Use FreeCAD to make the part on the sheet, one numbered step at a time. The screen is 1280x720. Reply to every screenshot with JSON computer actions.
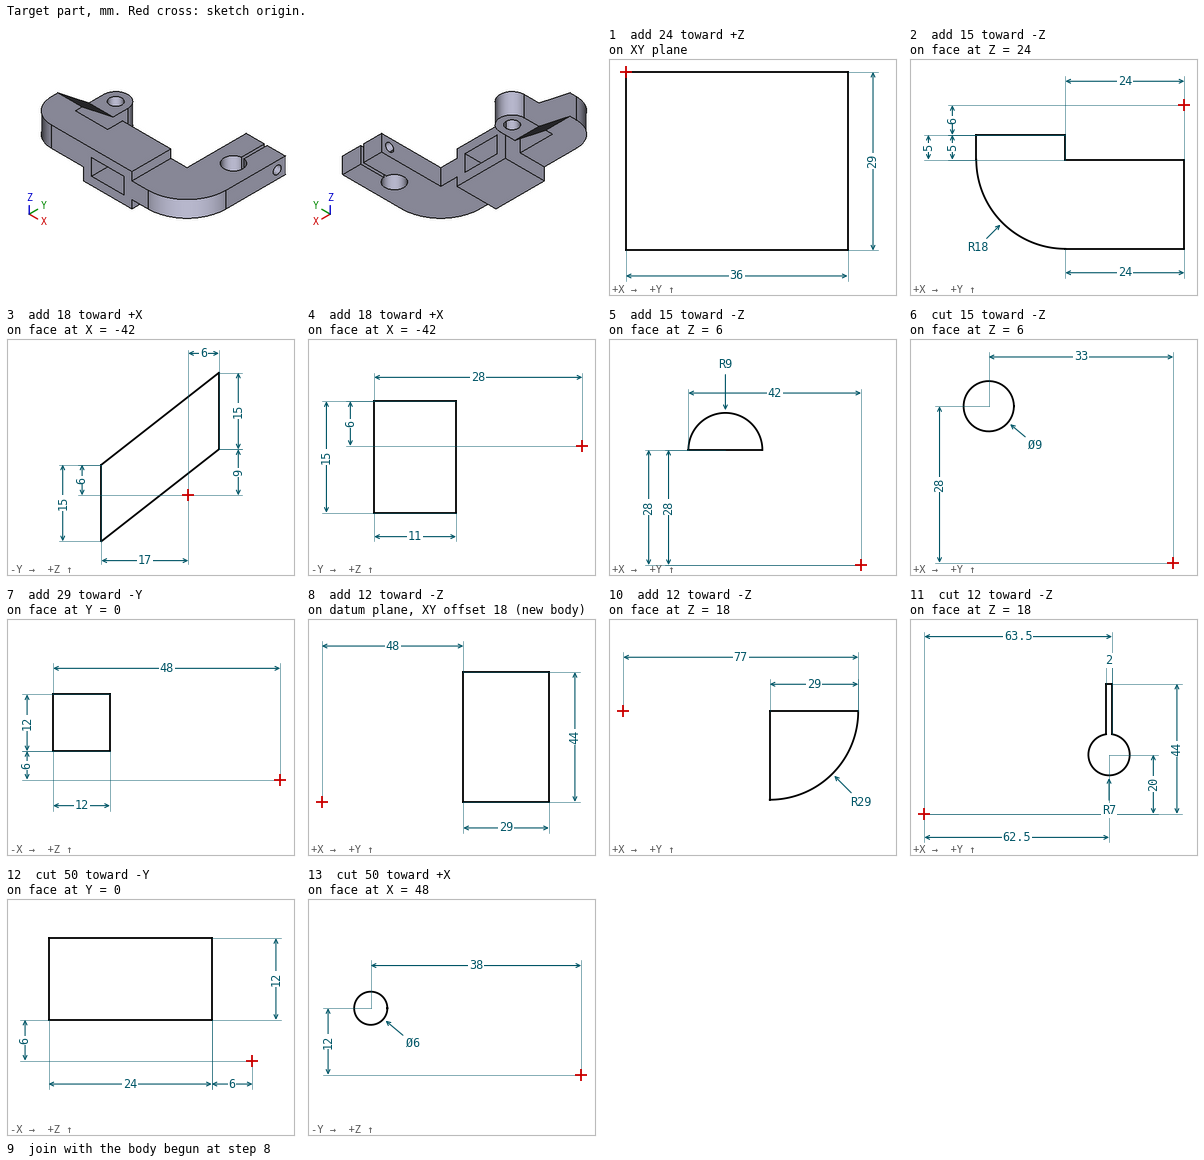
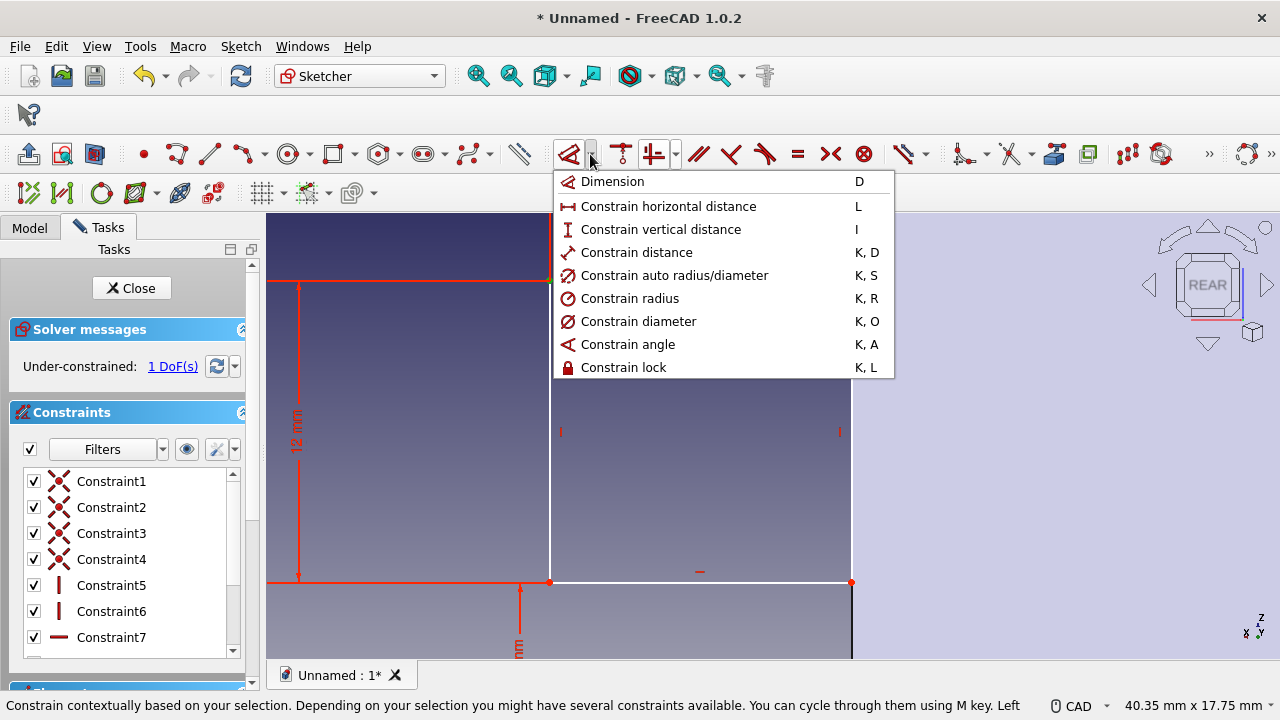
{"action": "left_click", "coordinate": [724, 206]}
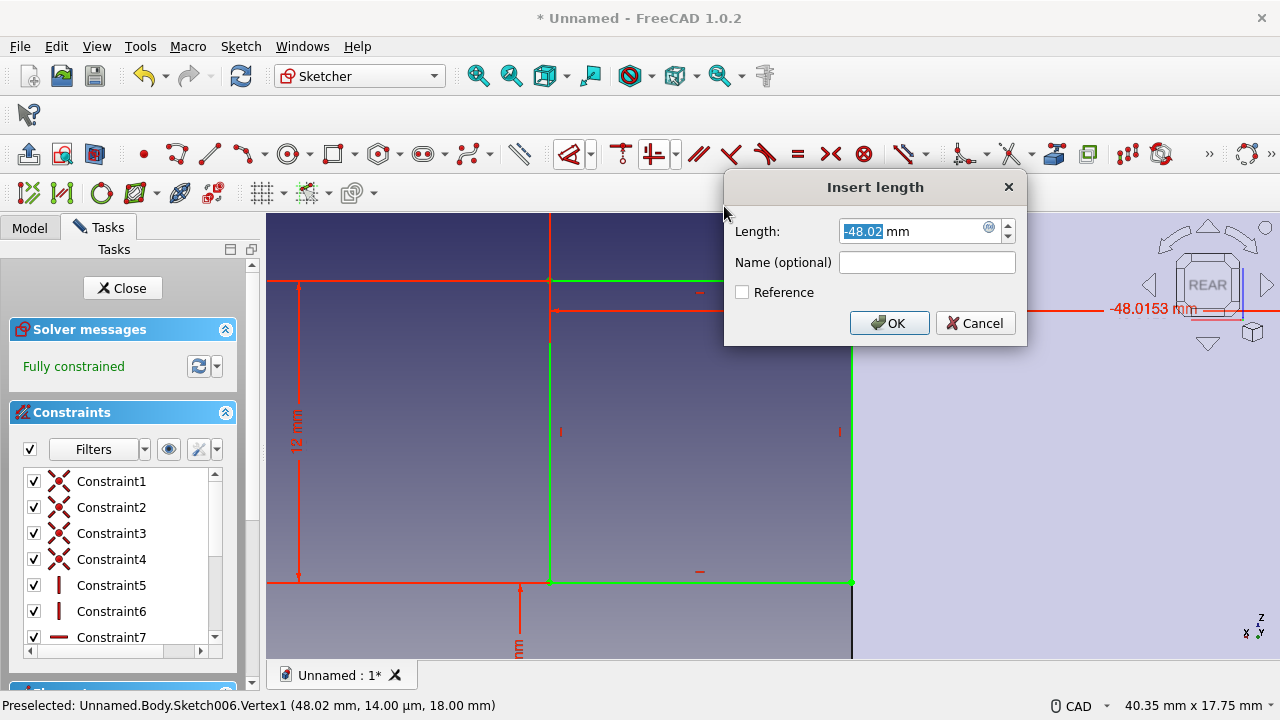
{"action": "type", "text": "-48"}
{"action": "key", "text": "Return"}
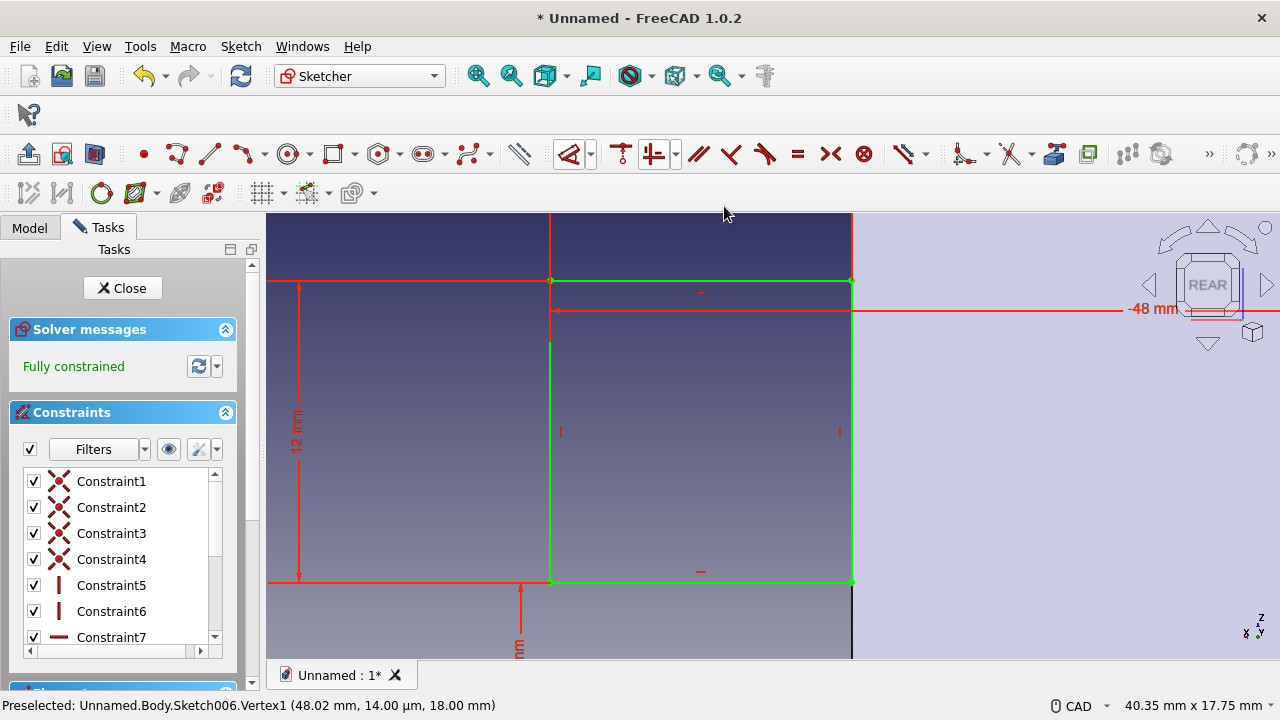
{"action": "left_click", "coordinate": [123, 288]}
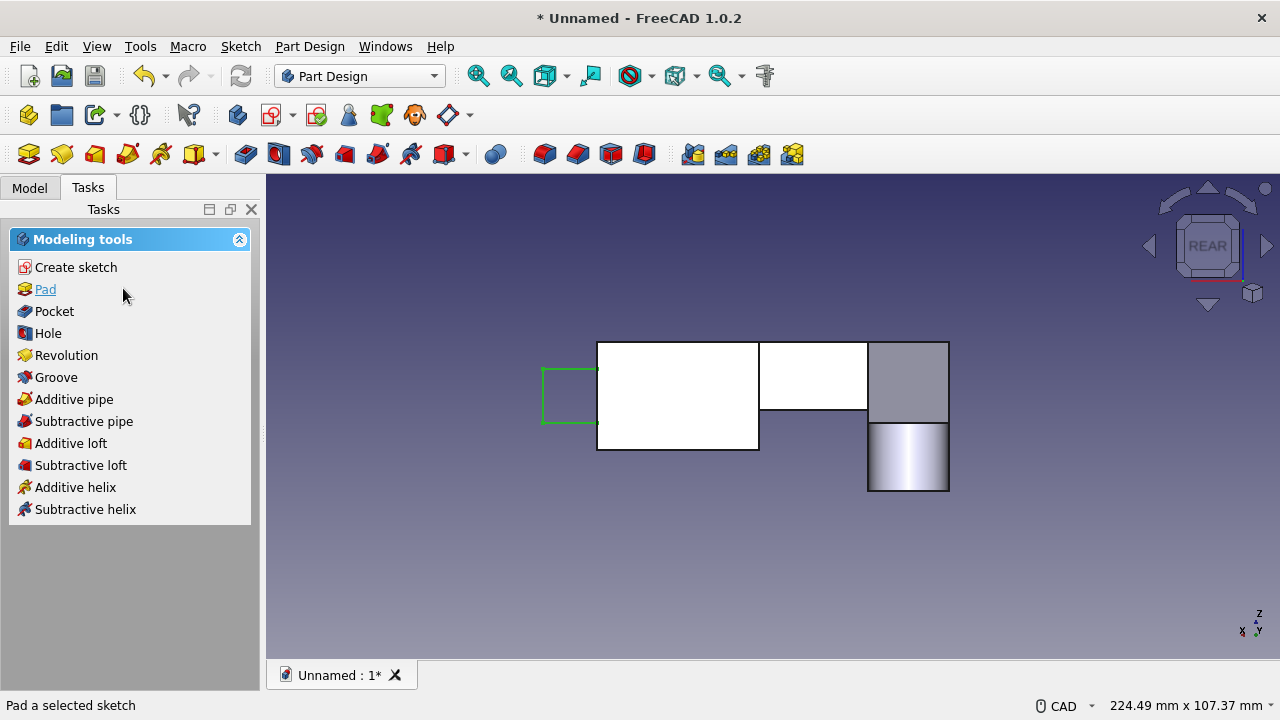
{"action": "left_click", "coordinate": [29, 154]}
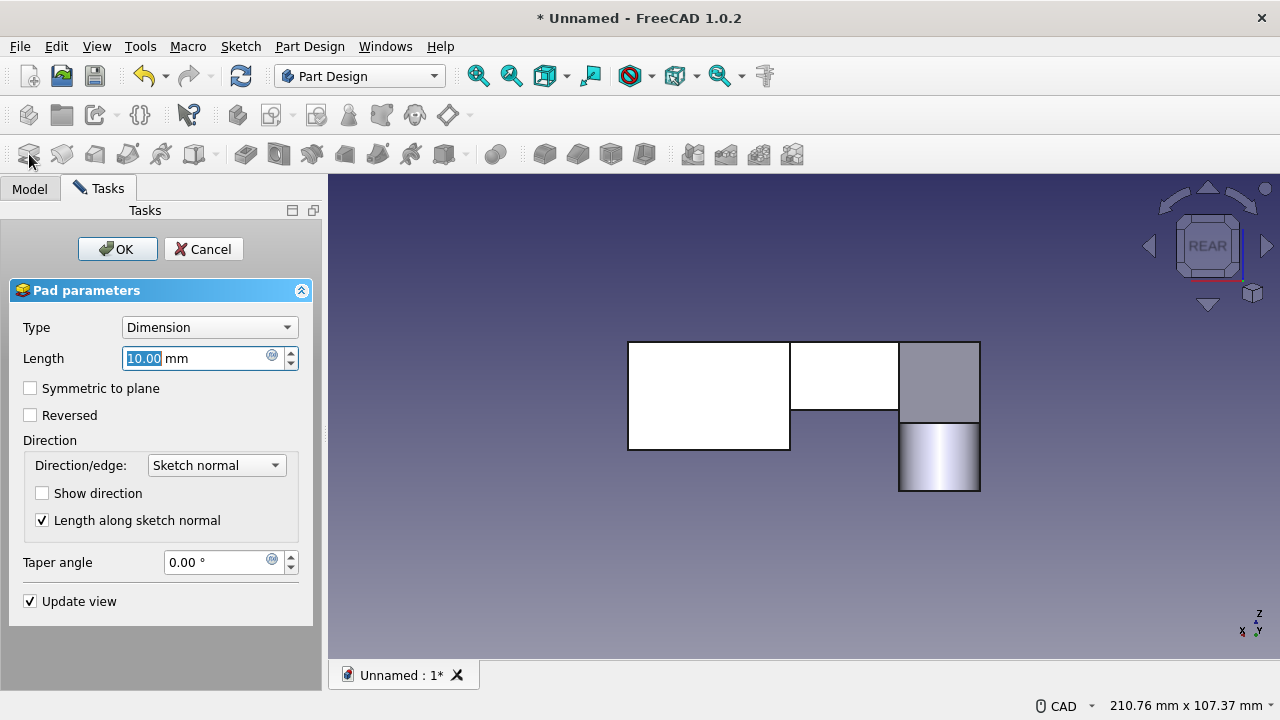
{"action": "type", "text": "29"}
{"action": "key", "text": "Tab"}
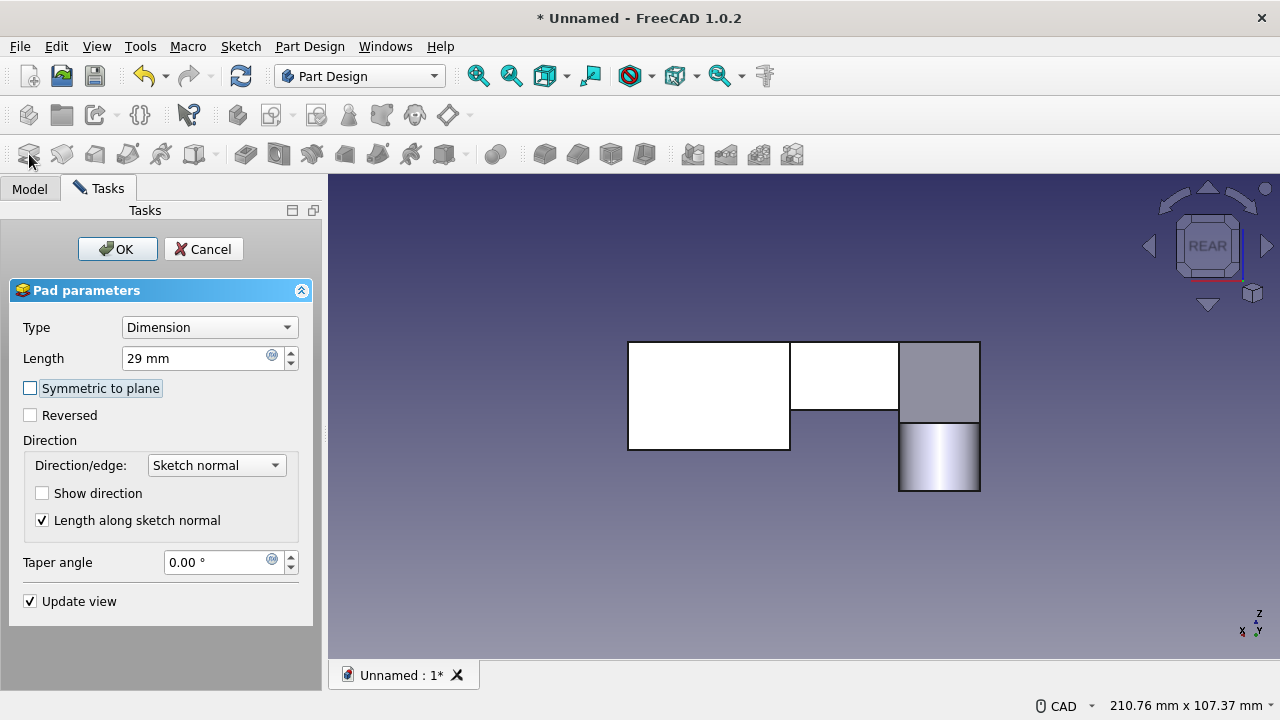
{"action": "left_click", "coordinate": [31, 415]}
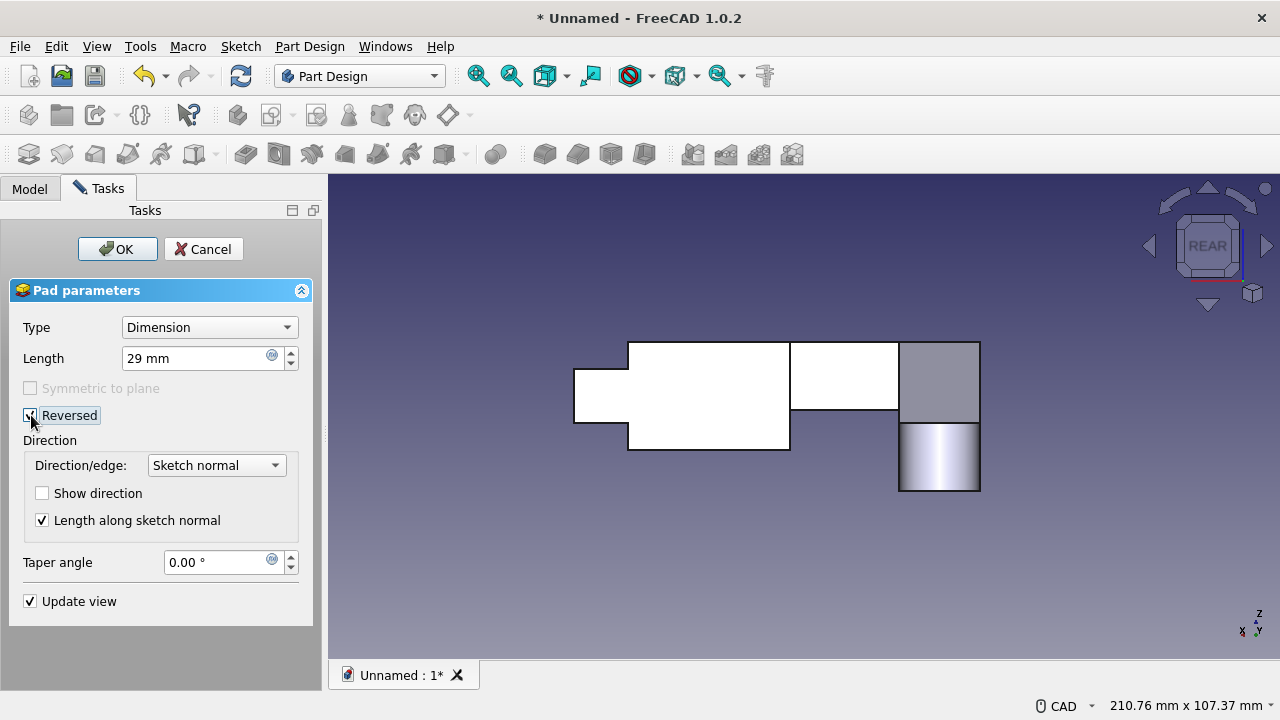
{"action": "left_click", "coordinate": [118, 249]}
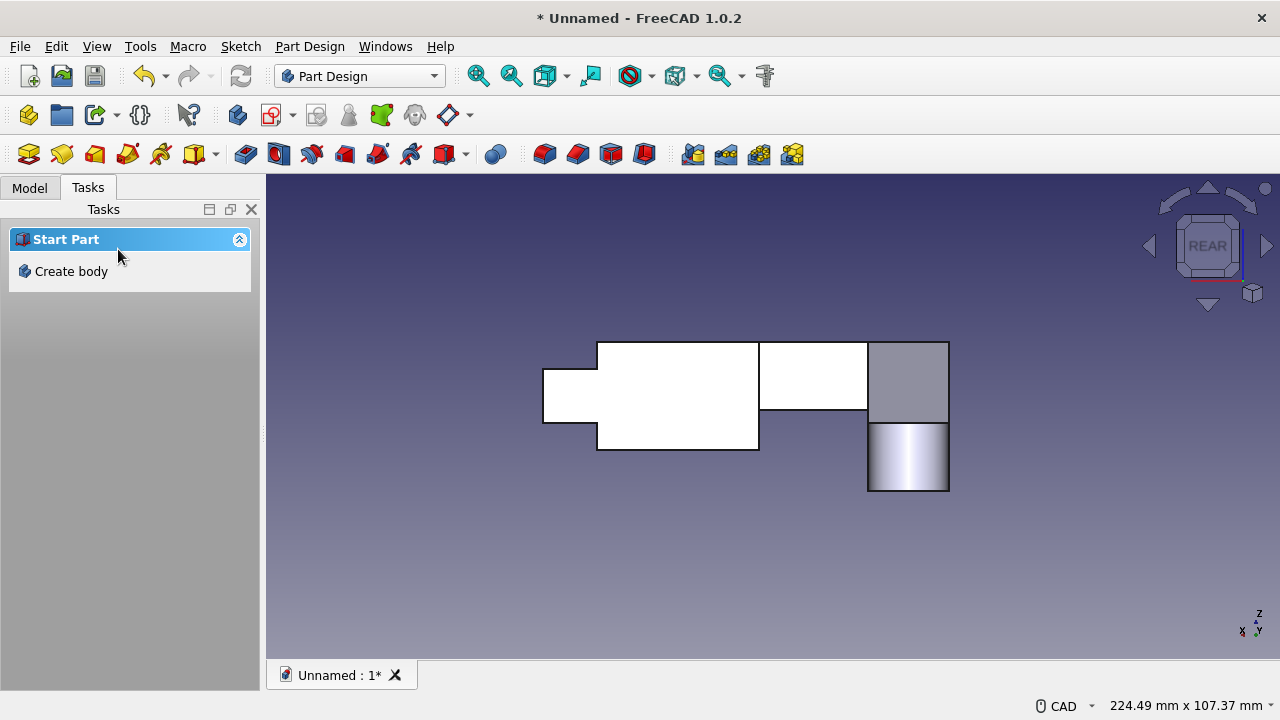
{"action": "key", "text": "v f"}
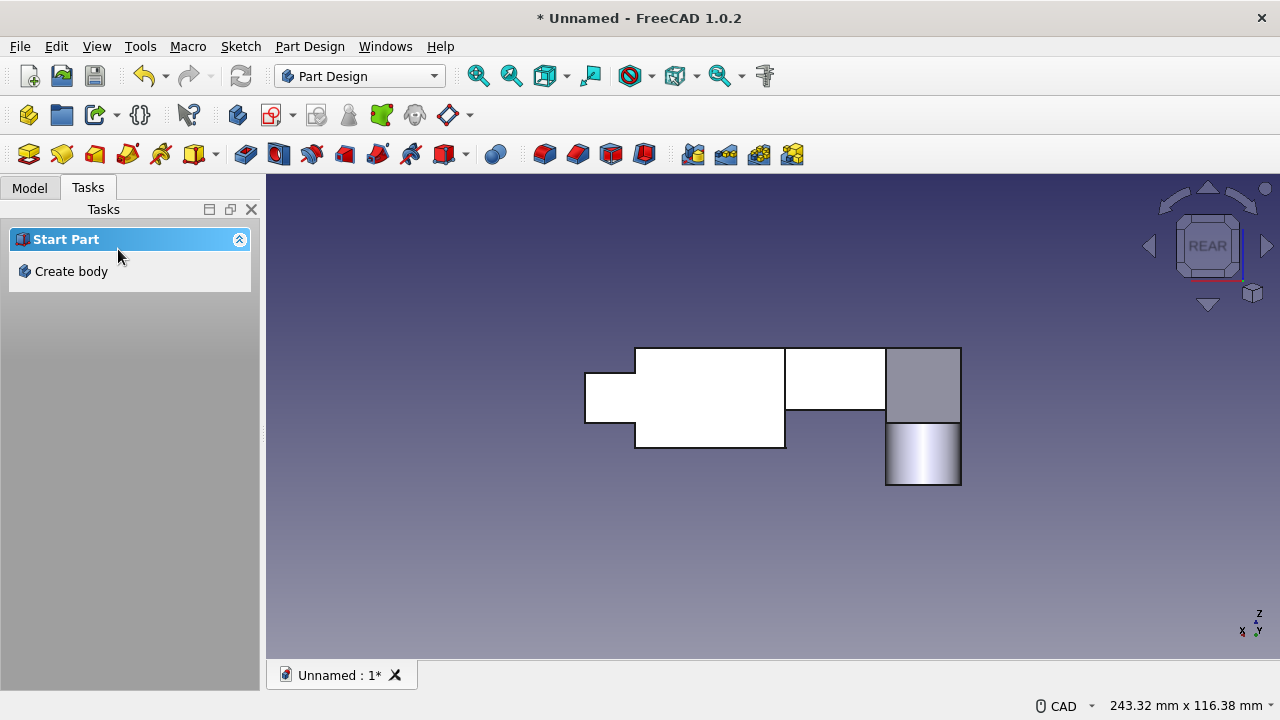
{"action": "left_click", "coordinate": [238, 116]}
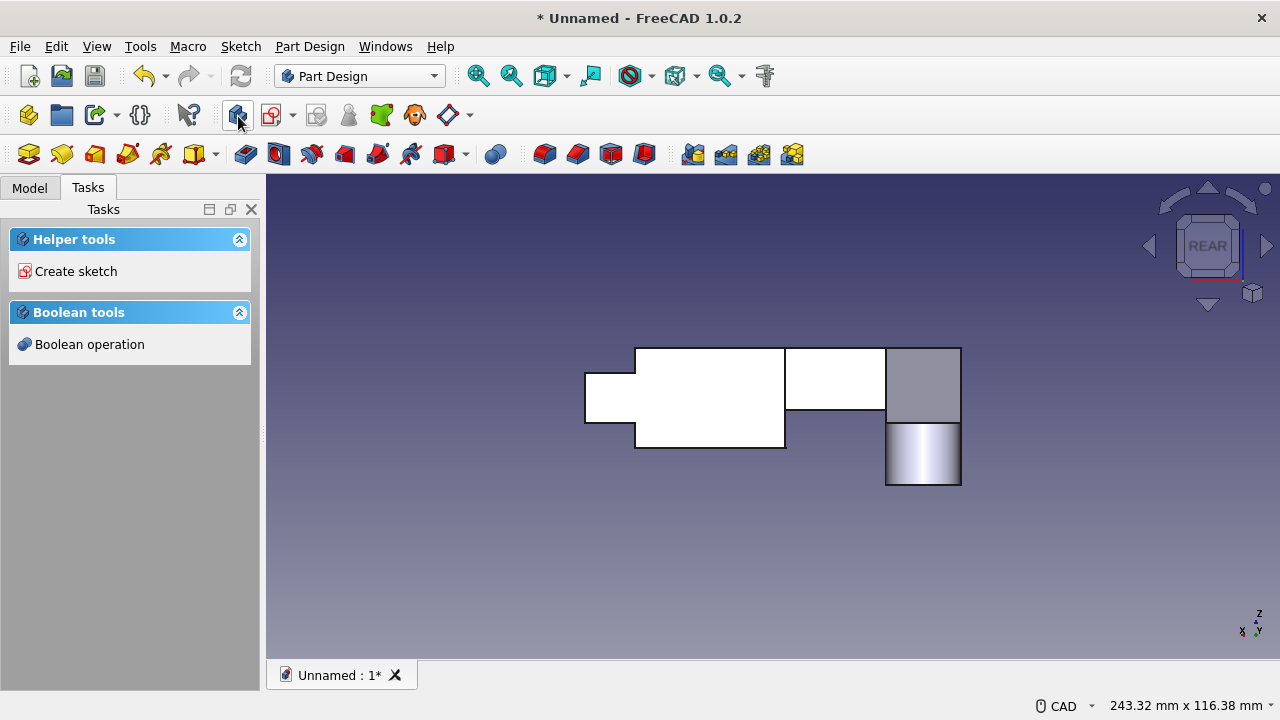
{"action": "left_click", "coordinate": [30, 188]}